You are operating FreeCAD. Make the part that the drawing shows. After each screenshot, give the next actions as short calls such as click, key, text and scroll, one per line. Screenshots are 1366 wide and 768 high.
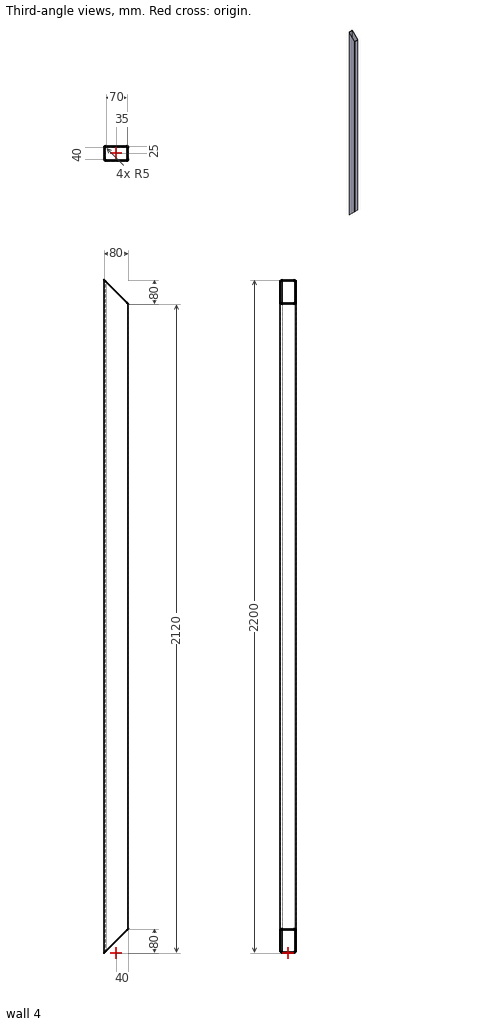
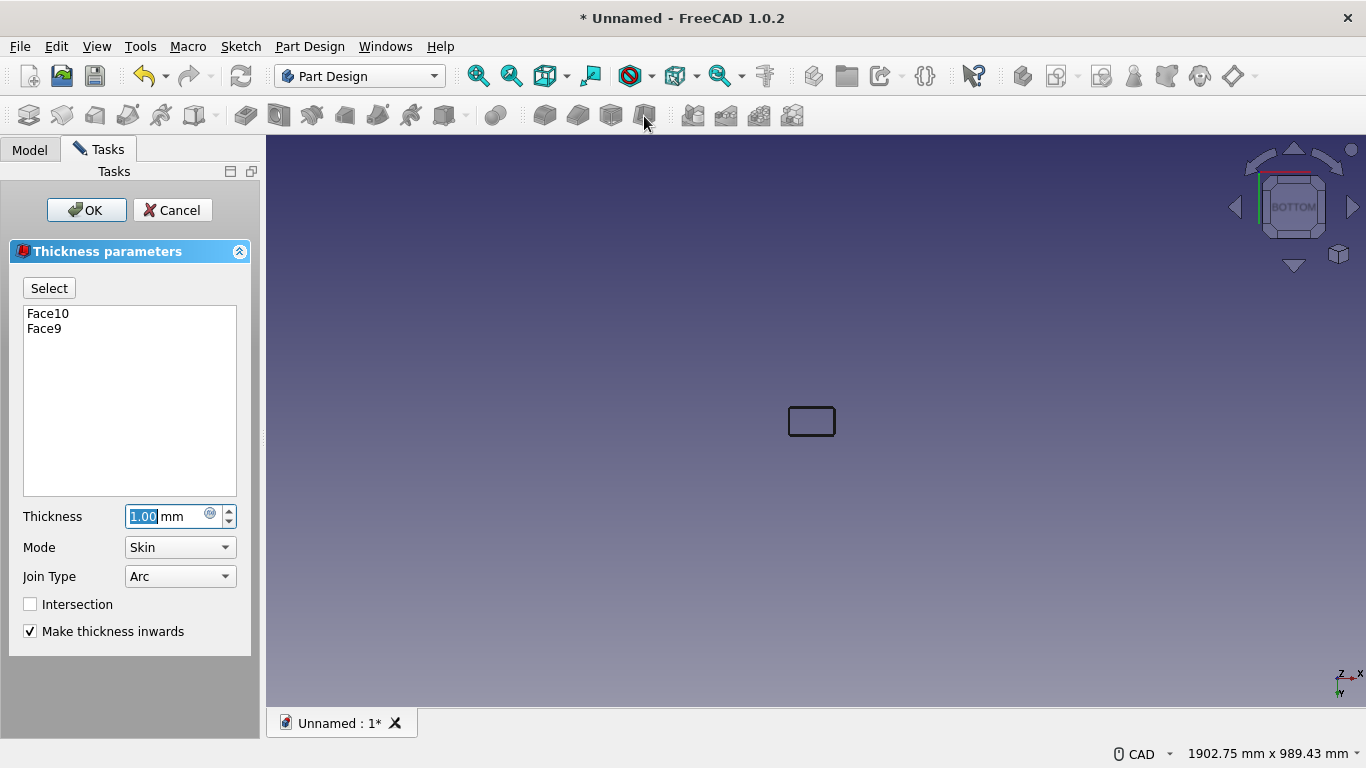
text(4)
key(Tab)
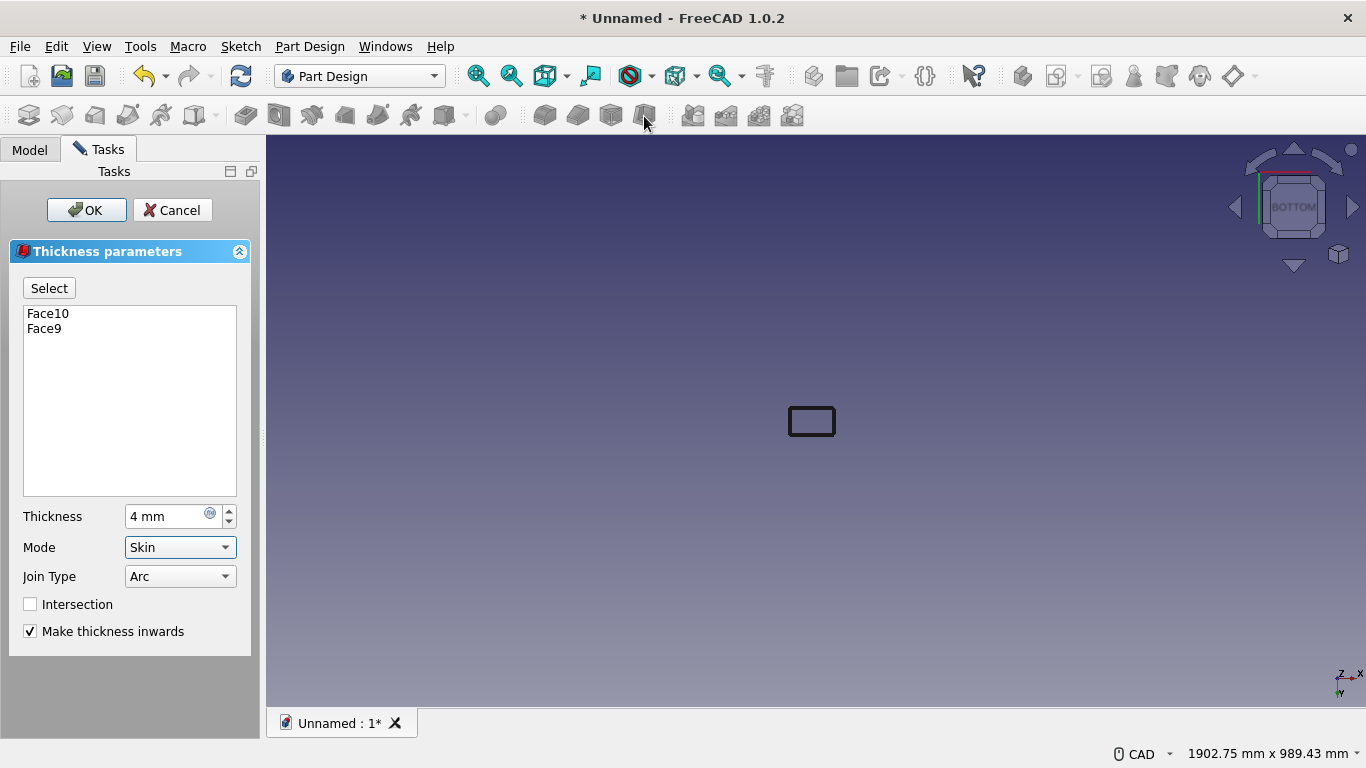
click(181, 576)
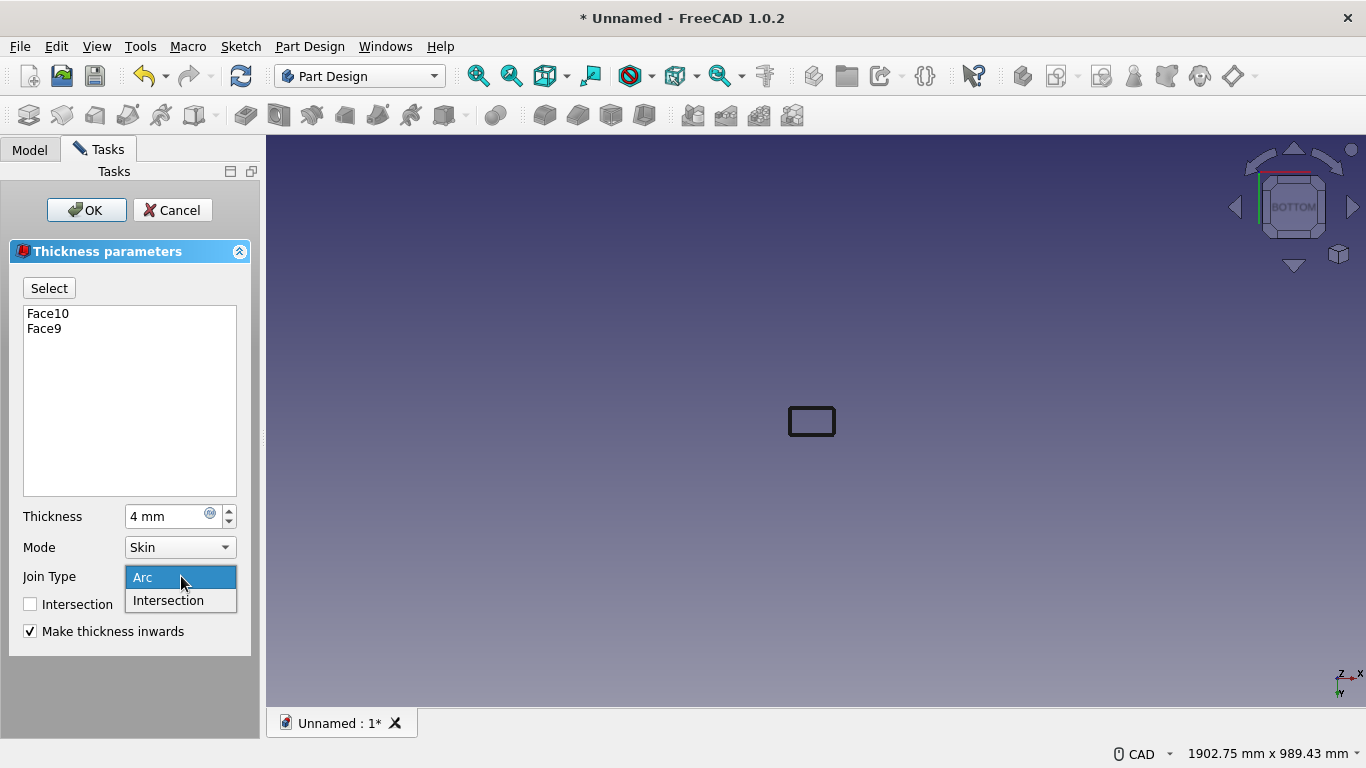
click(179, 600)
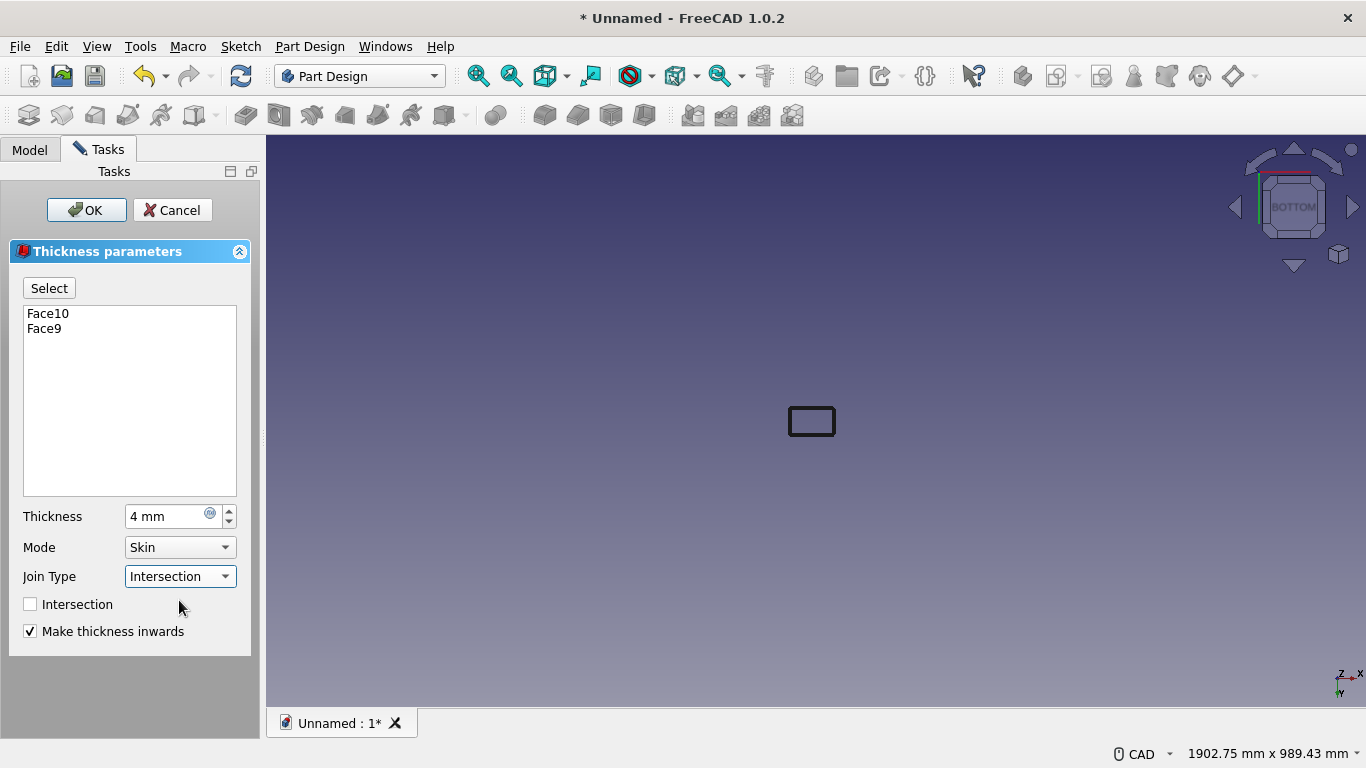
click(87, 210)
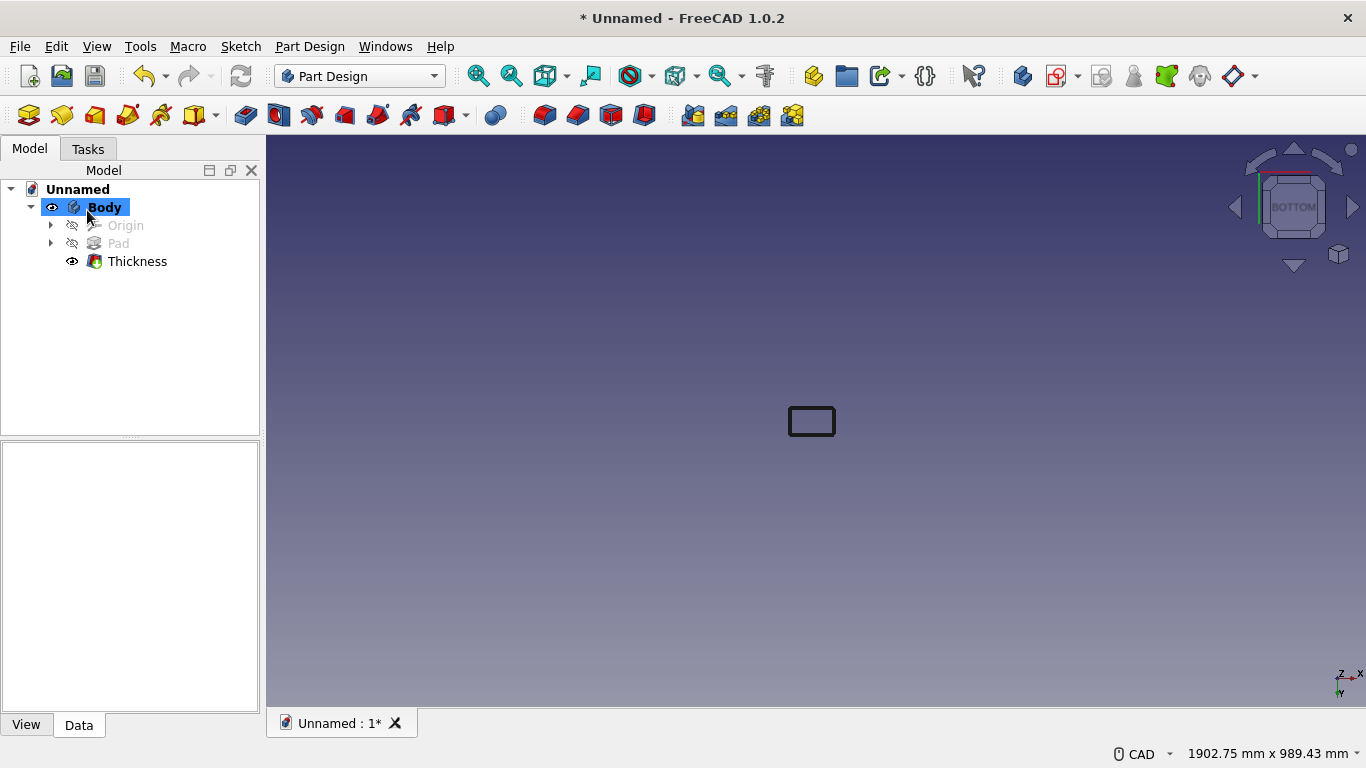
click(479, 76)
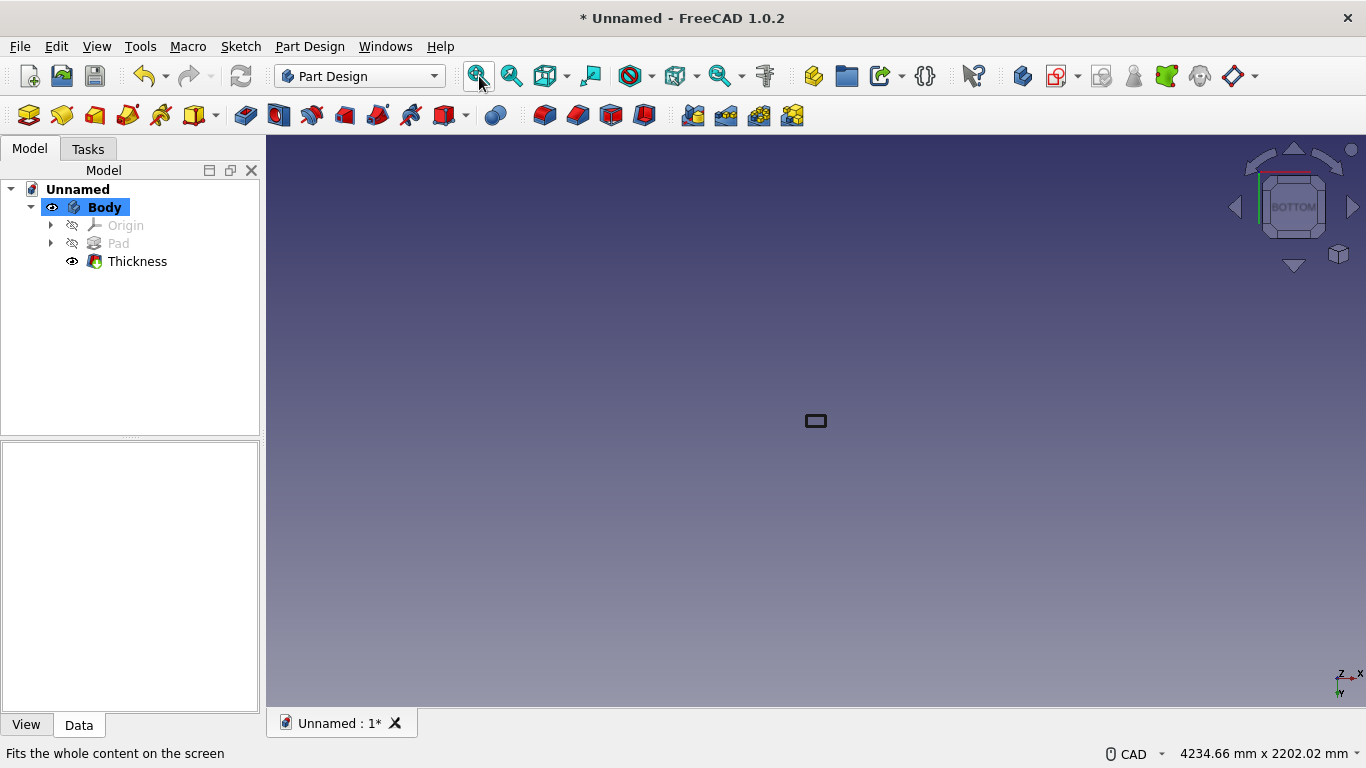
key(0)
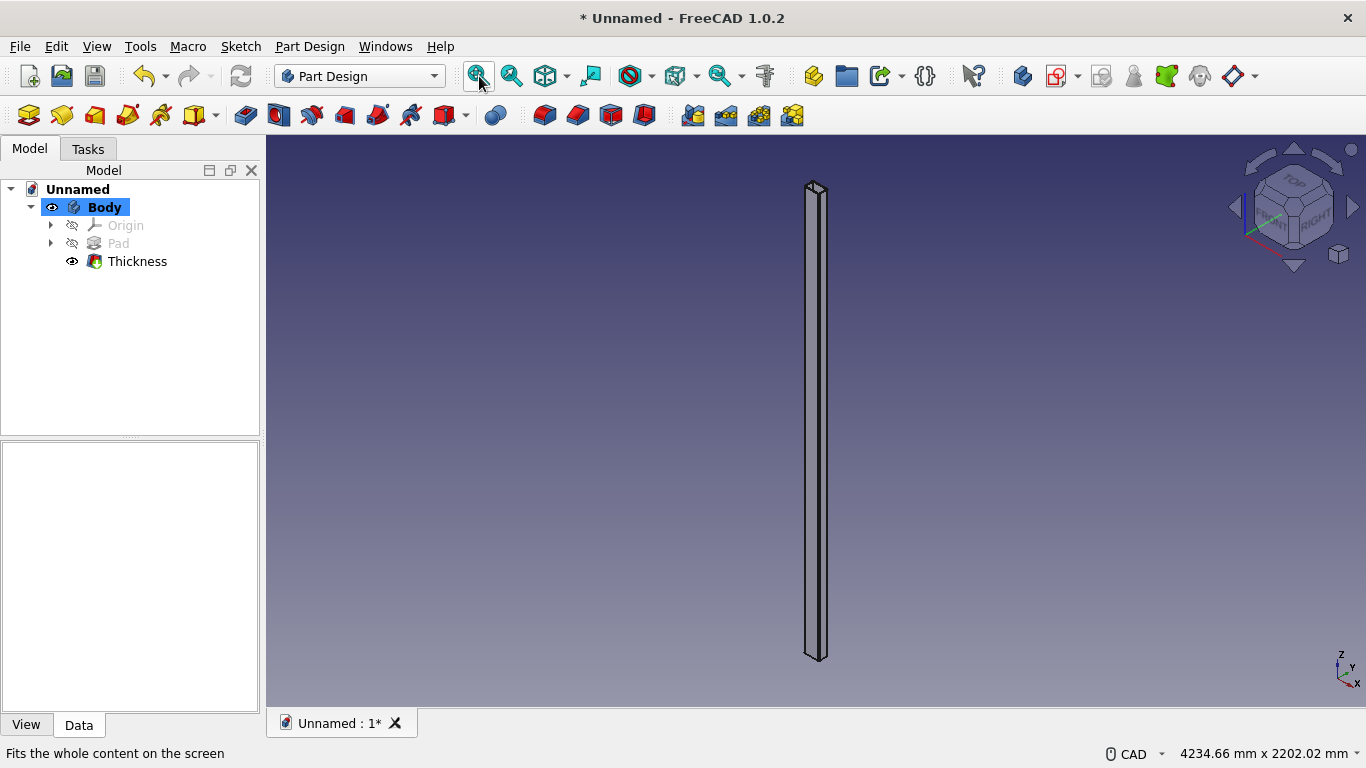
key(1)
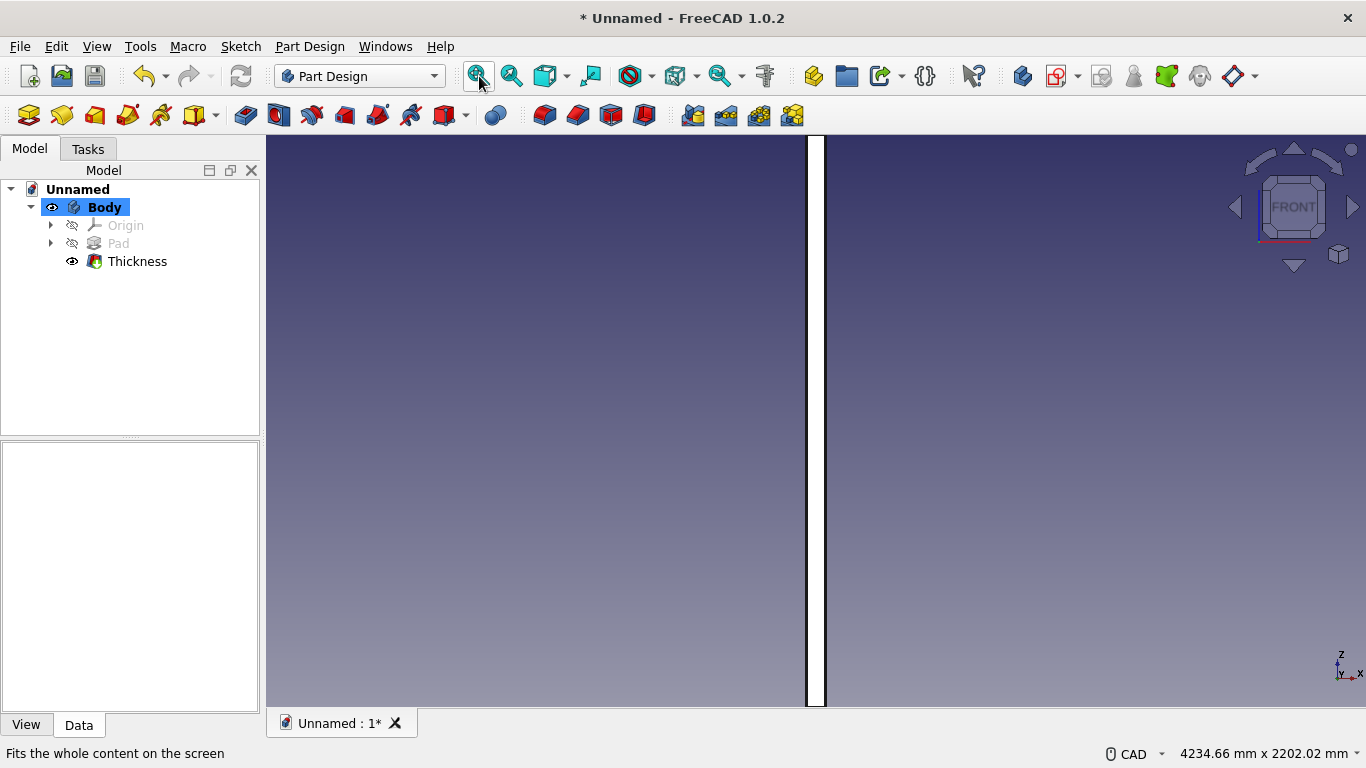
click(479, 76)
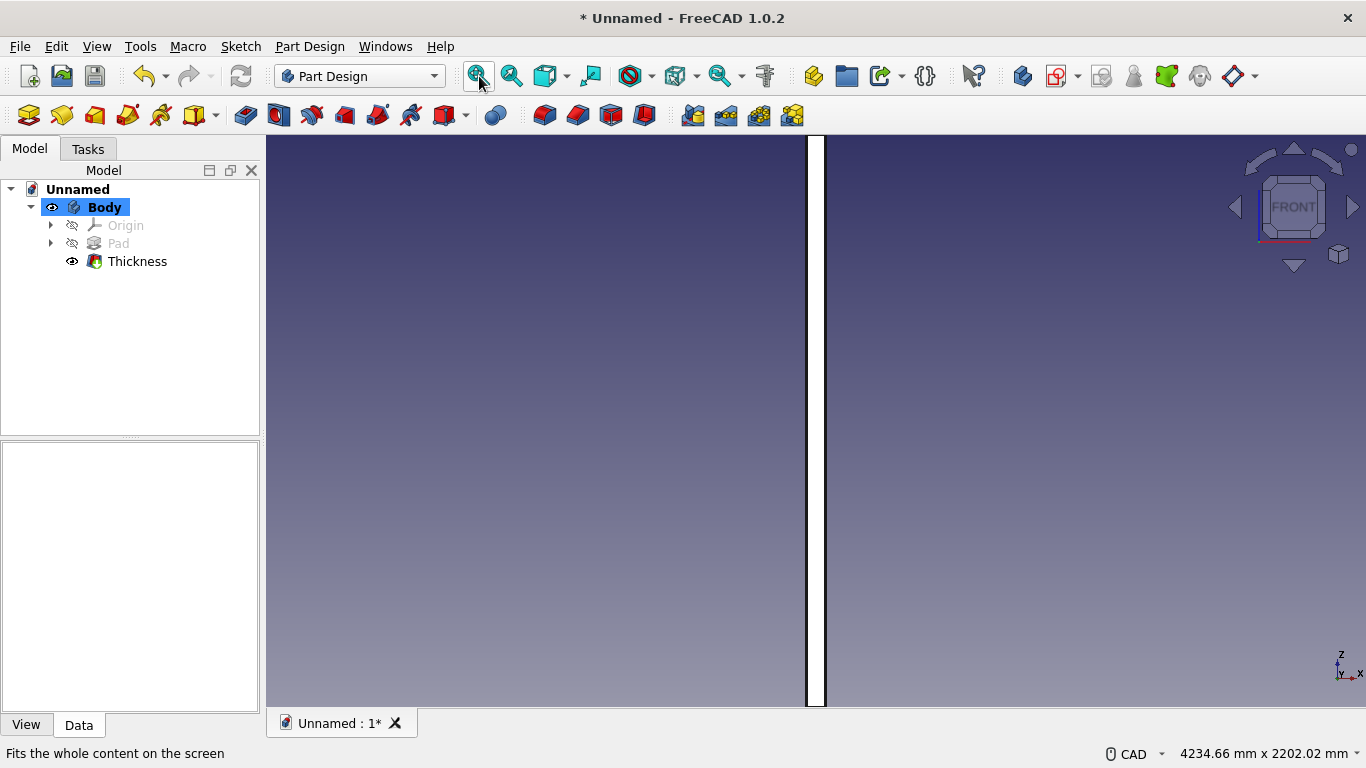
click(816, 175)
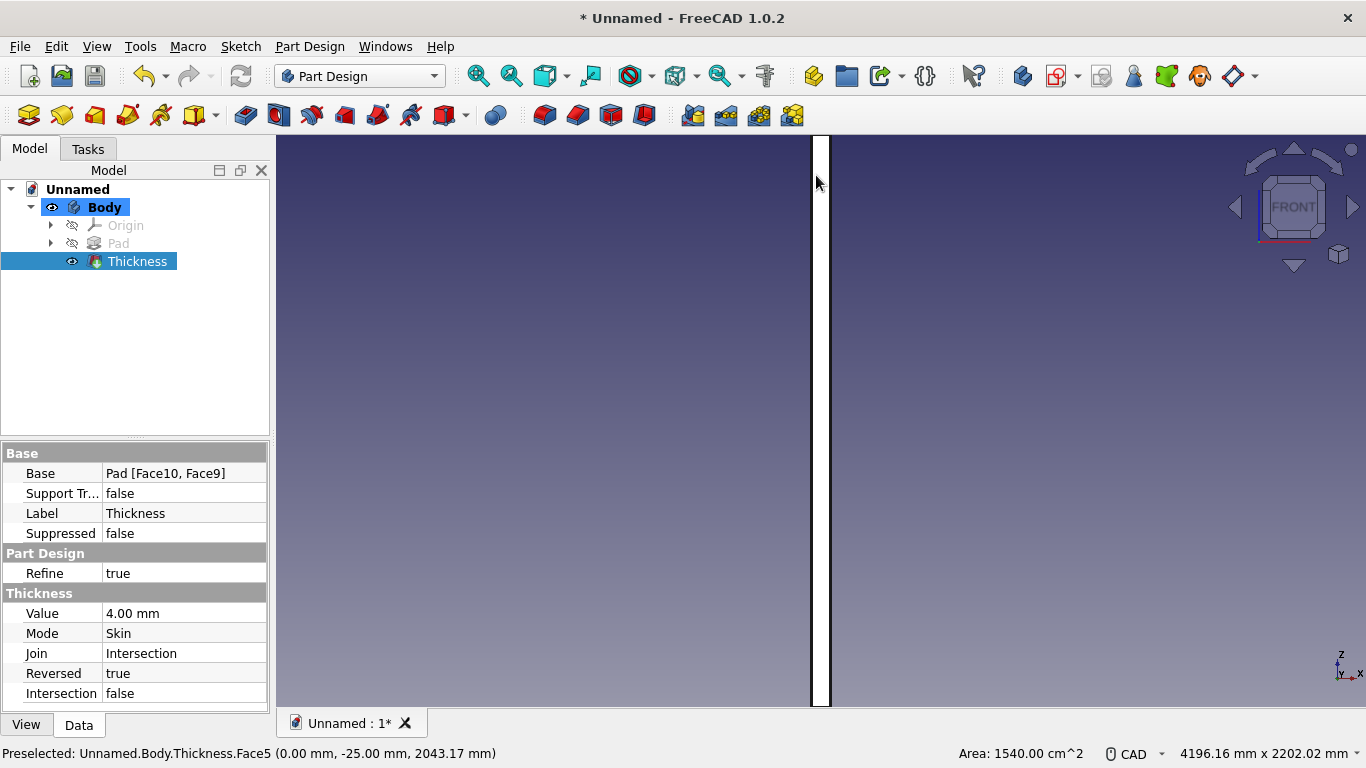
click(1056, 76)